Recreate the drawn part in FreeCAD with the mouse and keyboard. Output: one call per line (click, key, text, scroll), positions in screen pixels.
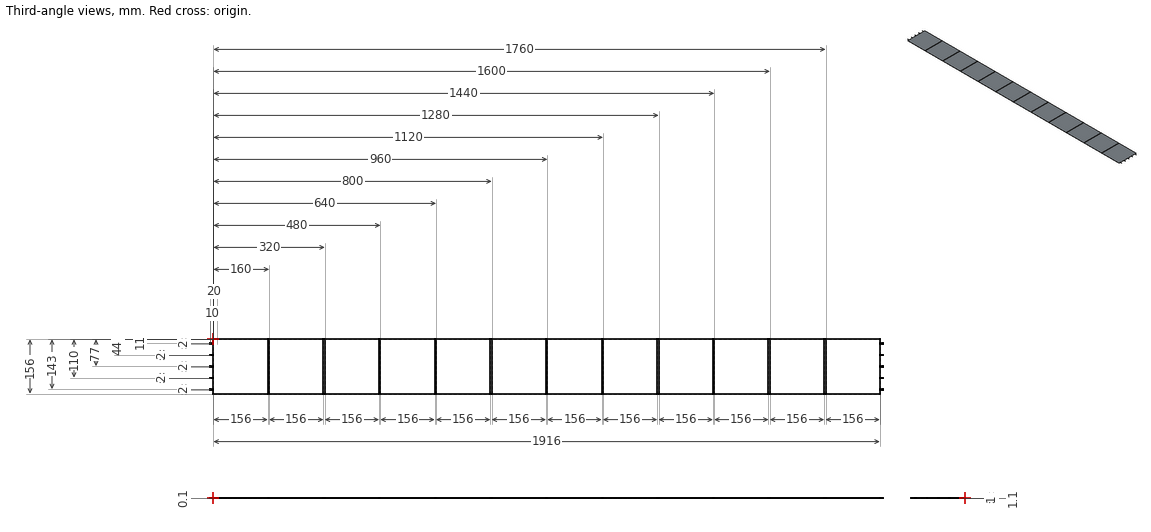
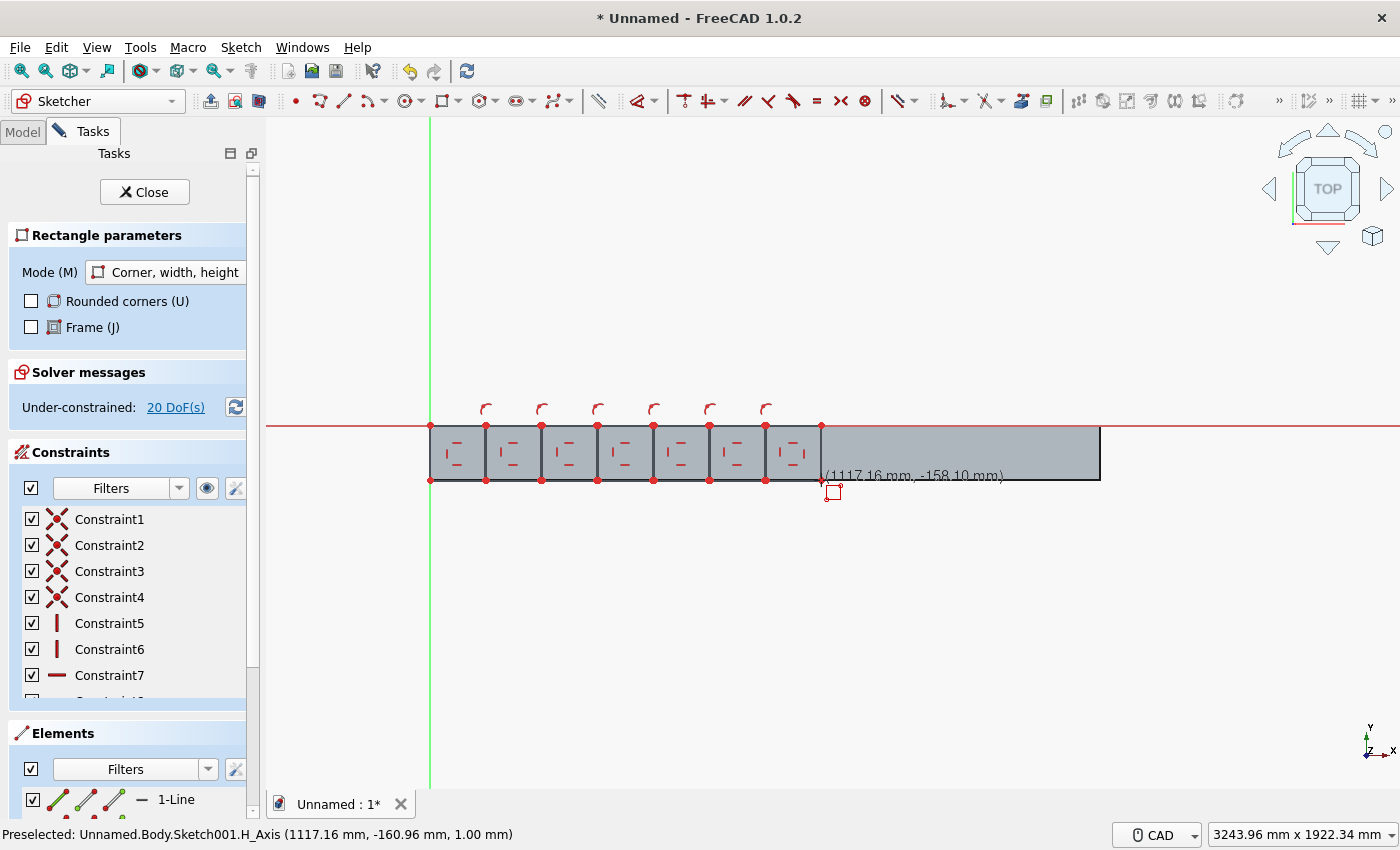
scroll(822, 426, up, 13)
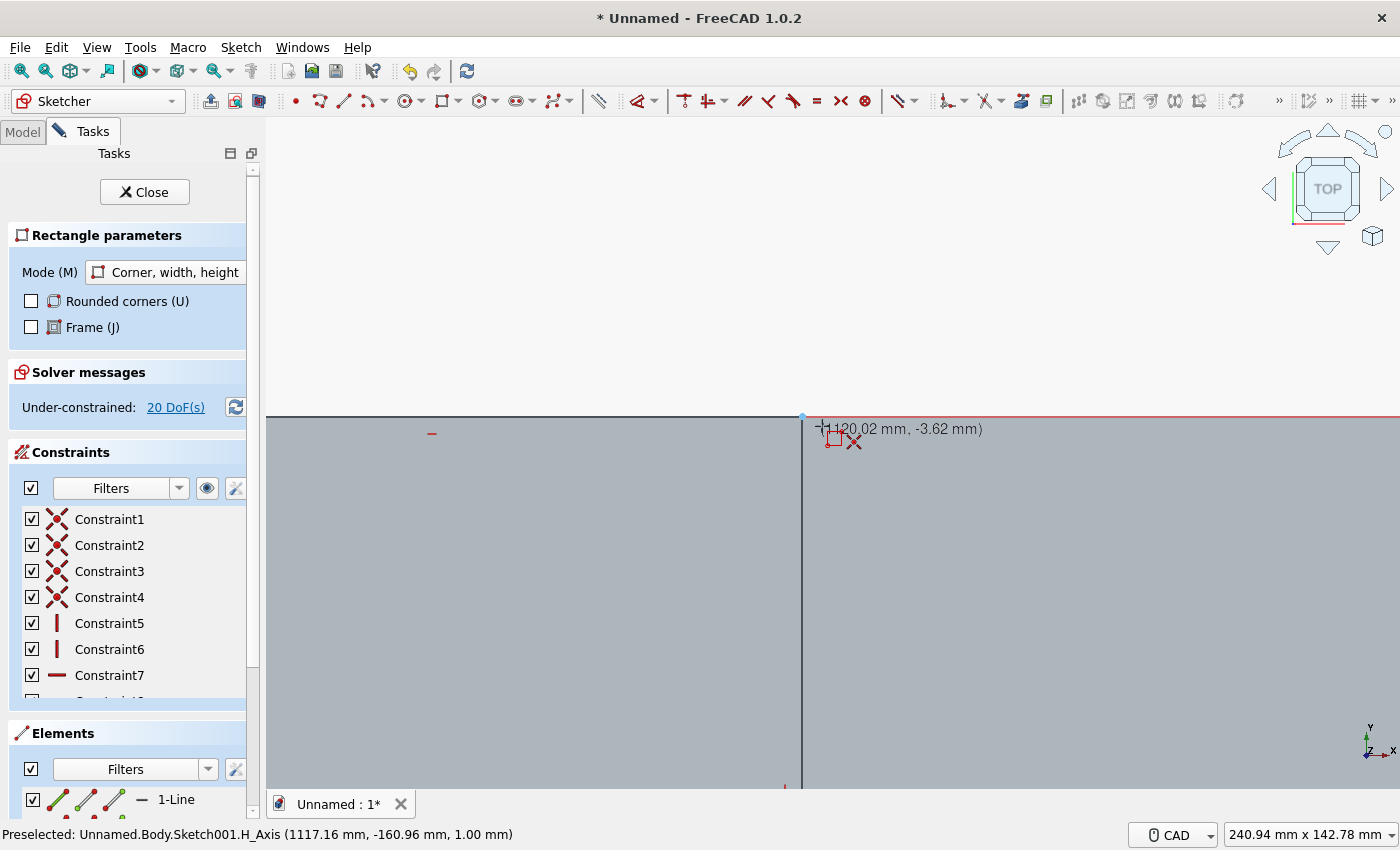
click(816, 417)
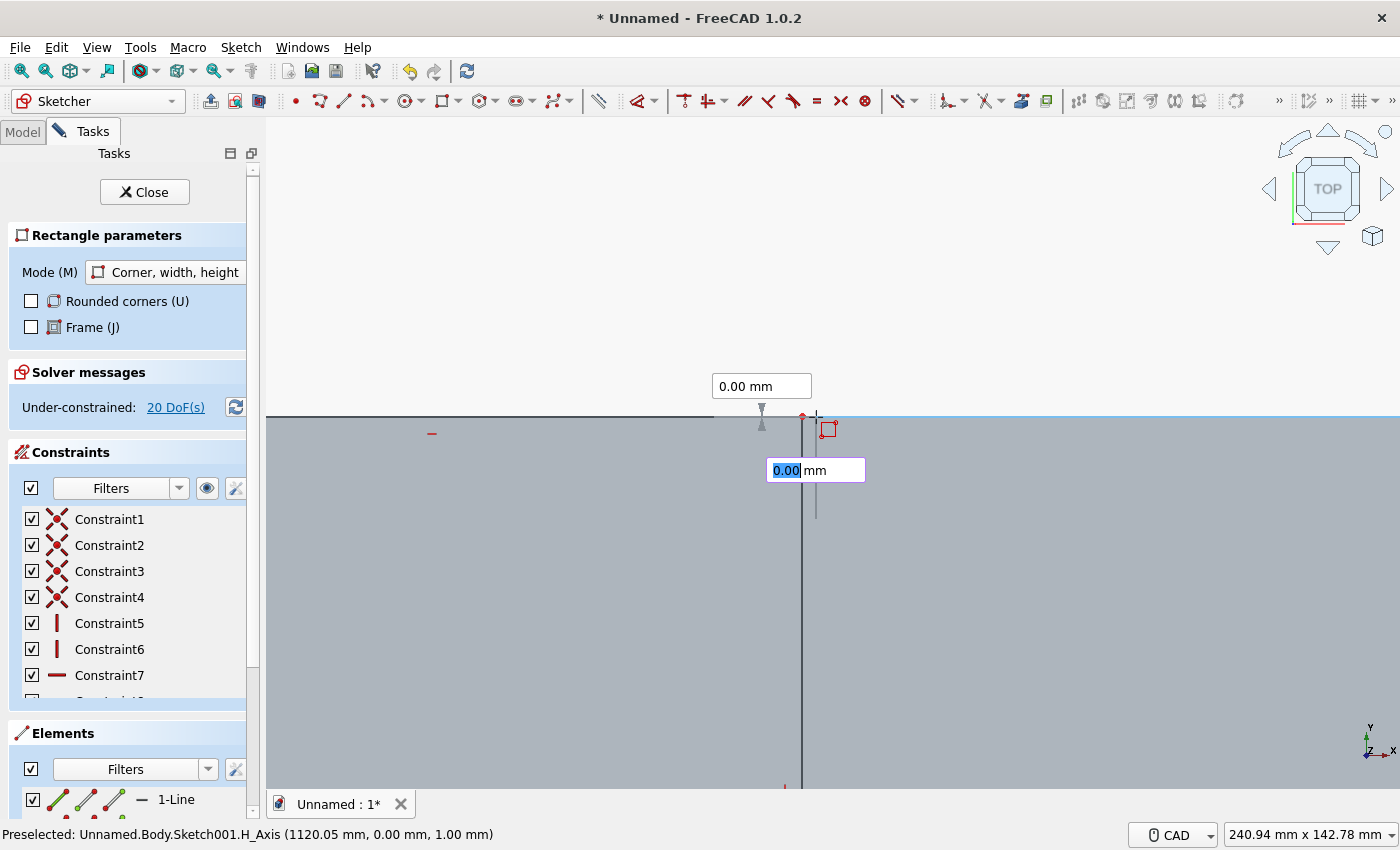
scroll(822, 426, down, 13)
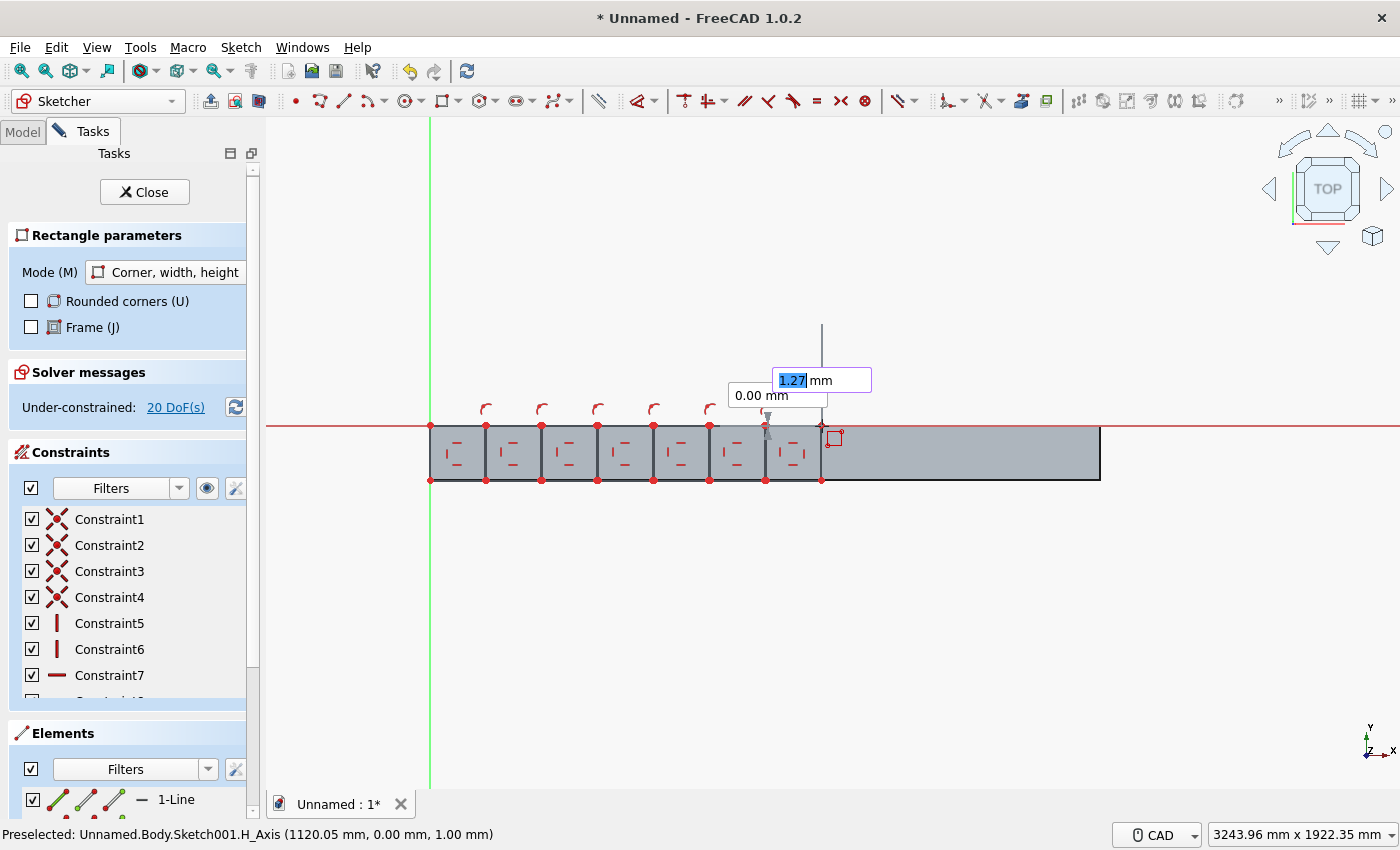
click(877, 480)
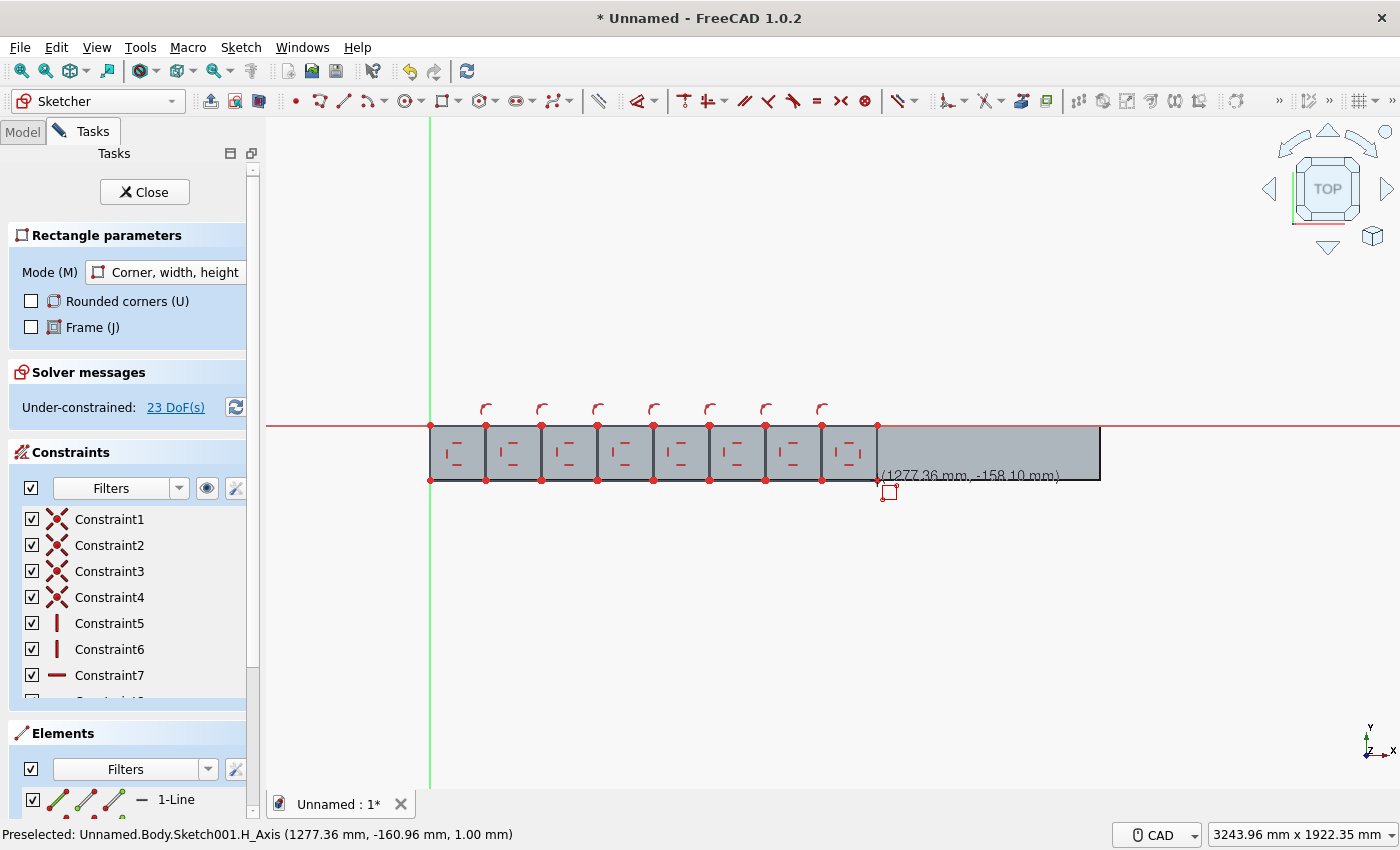
scroll(878, 426, up, 13)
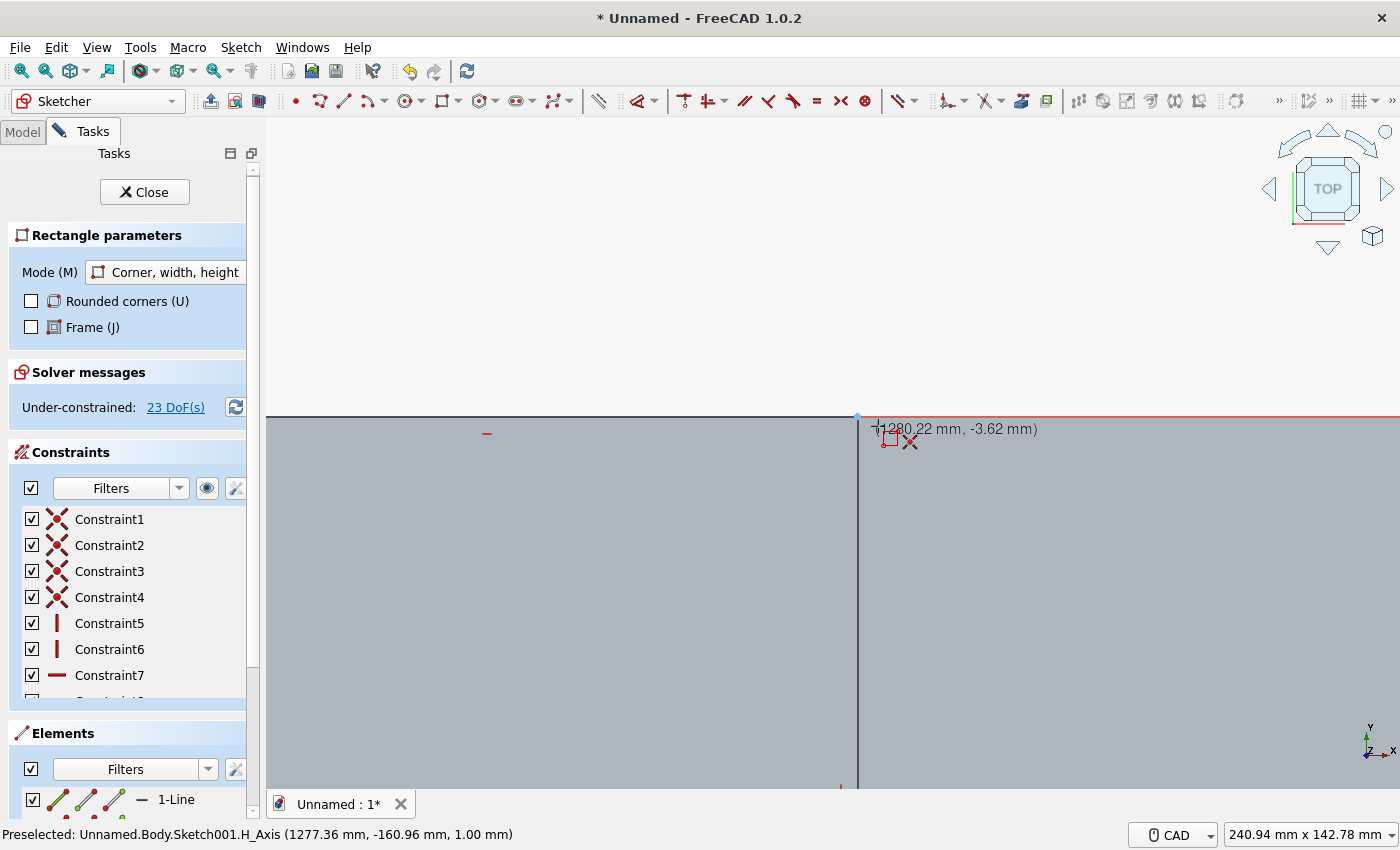
click(870, 417)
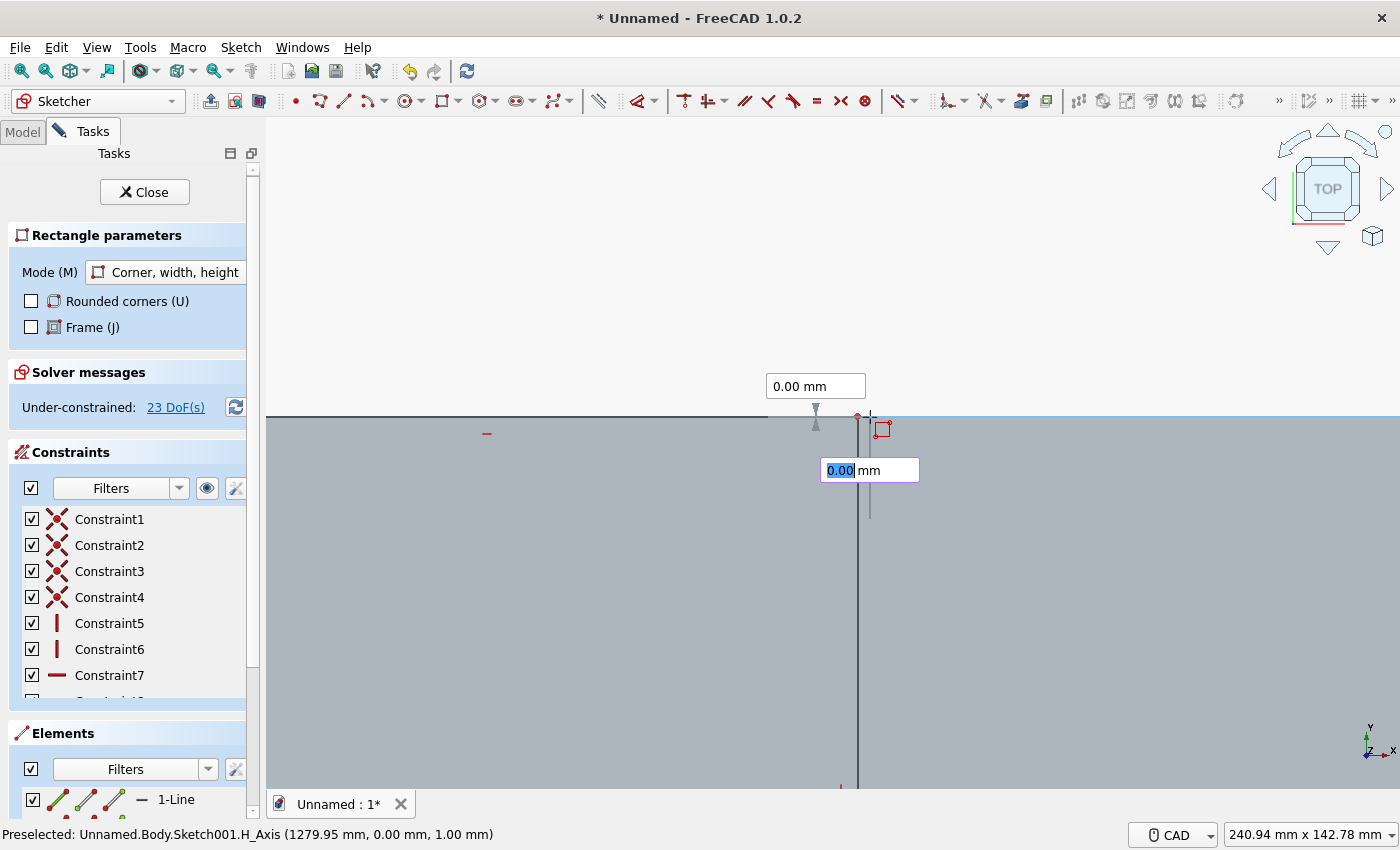
scroll(878, 426, down, 13)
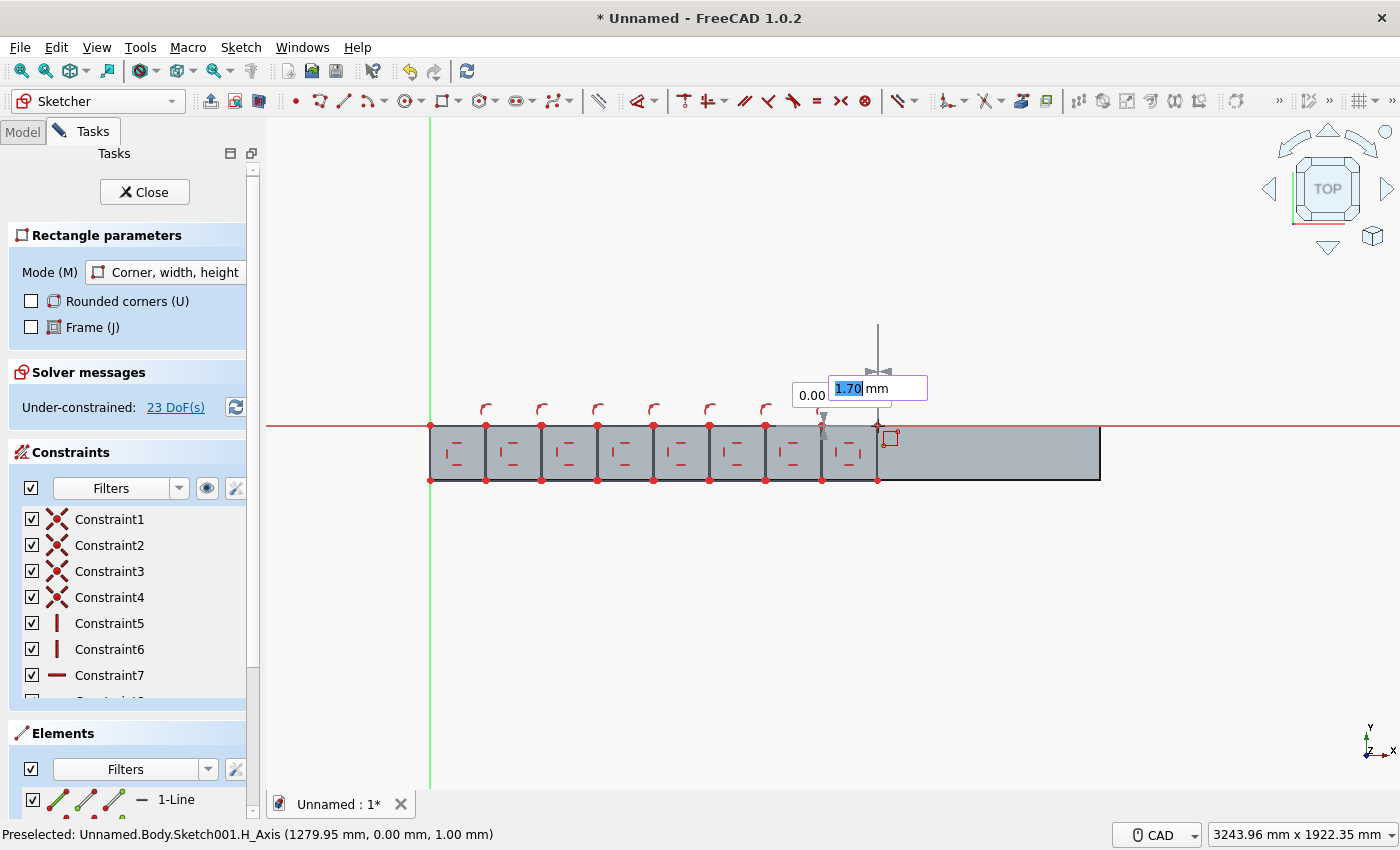
click(932, 480)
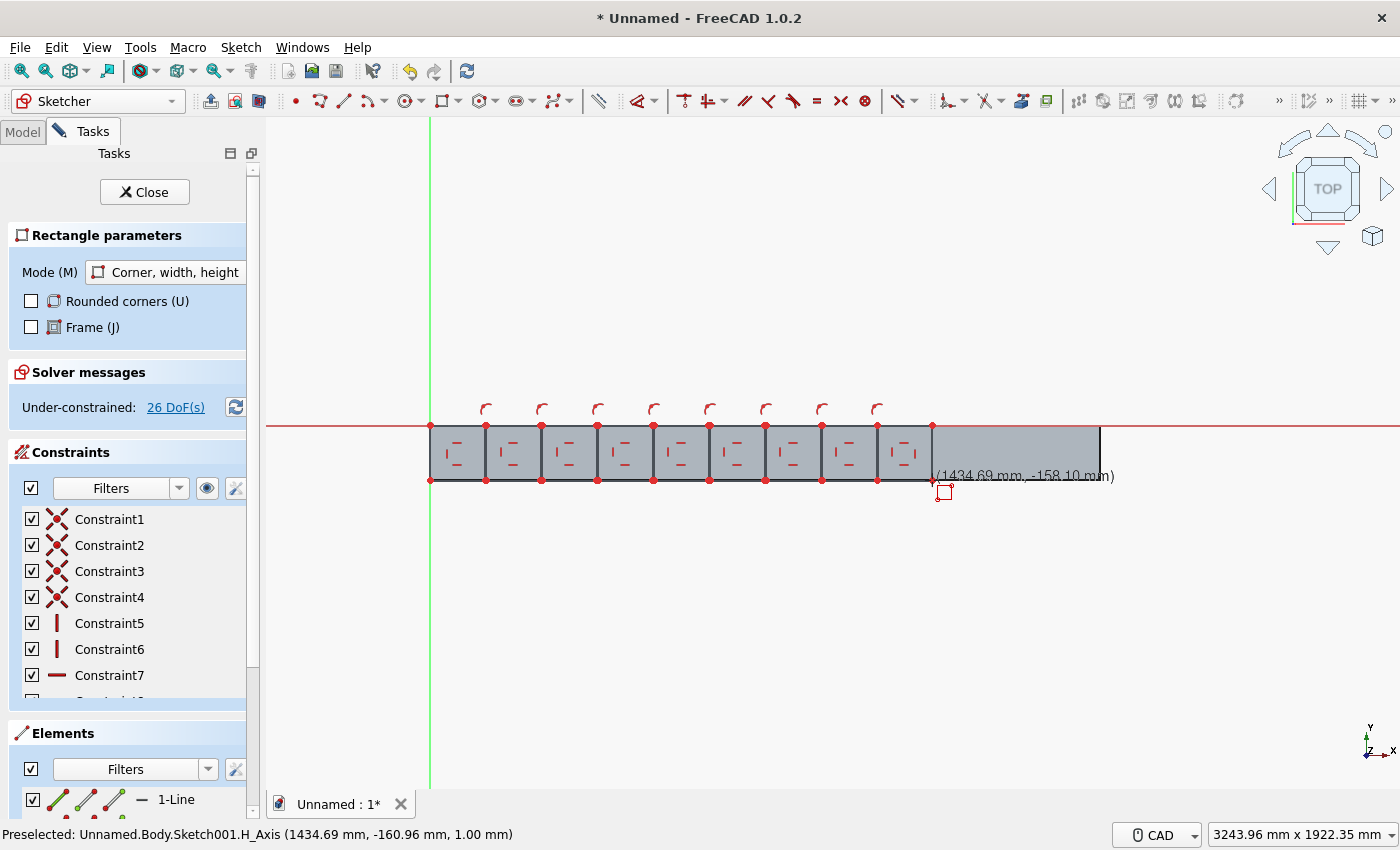
scroll(934, 426, up, 13)